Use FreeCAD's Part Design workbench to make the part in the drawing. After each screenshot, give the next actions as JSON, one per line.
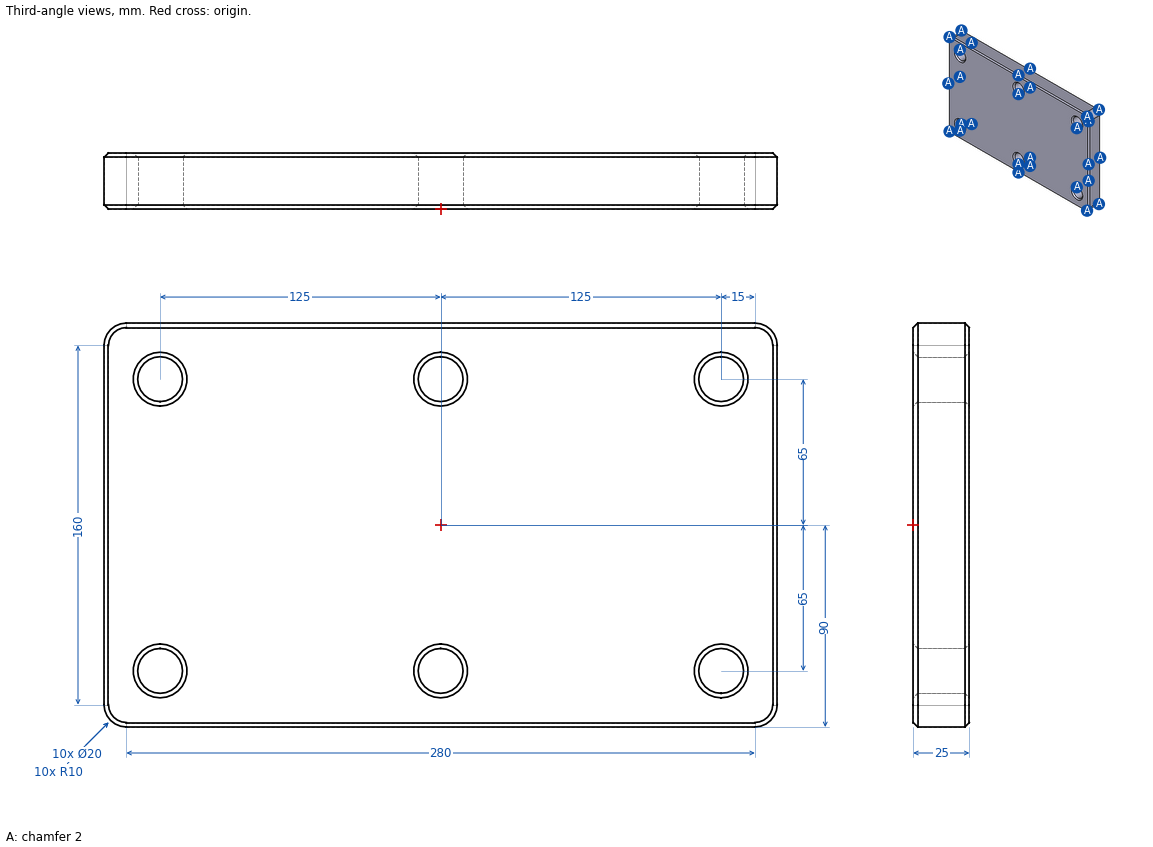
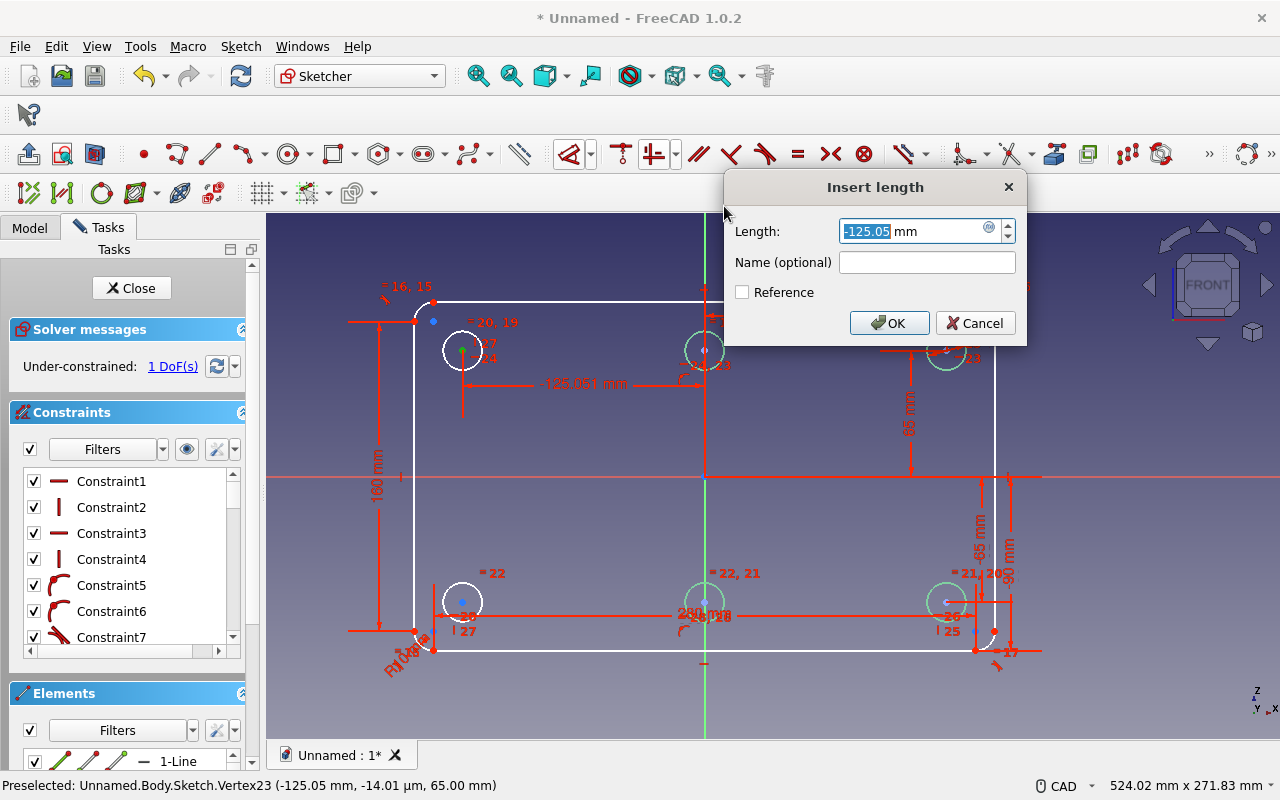
{"action": "type", "text": "-125"}
{"action": "key", "text": "Return"}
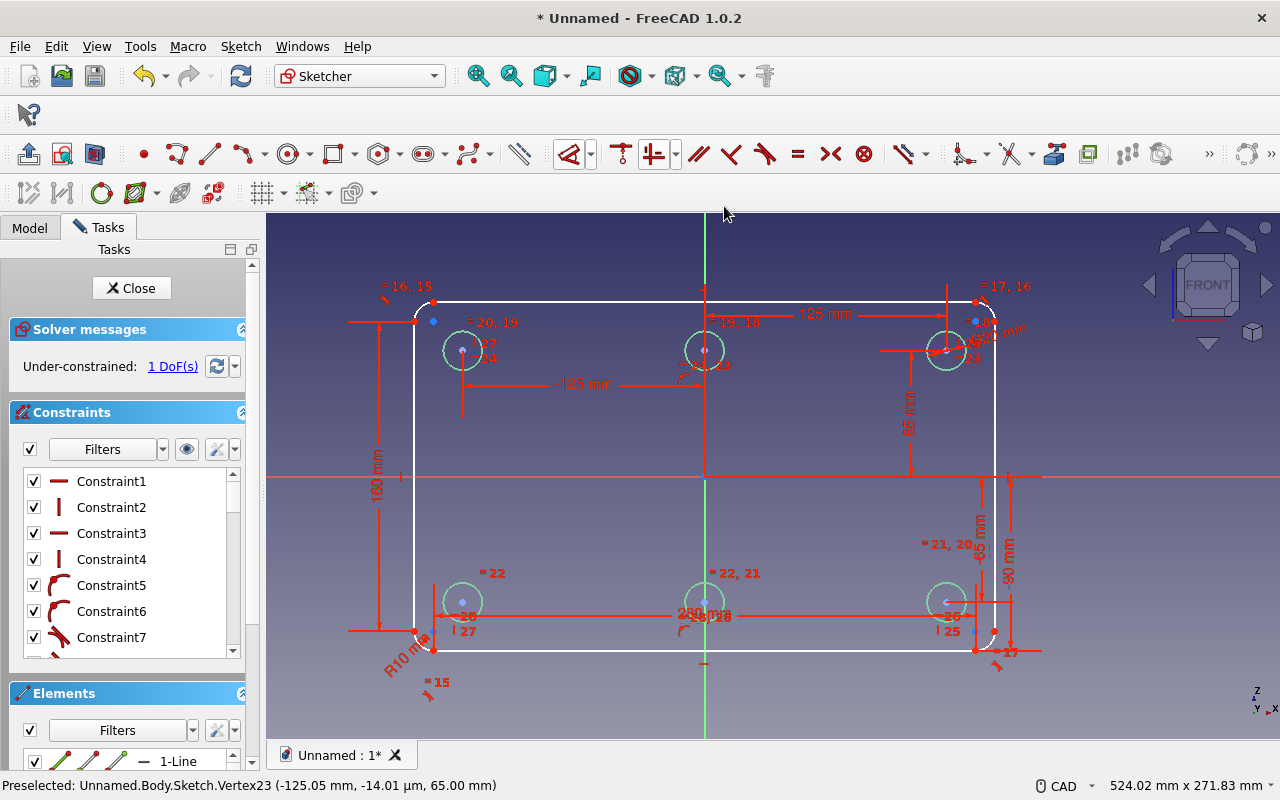
{"action": "scroll", "coordinate": [976, 302], "scroll_direction": "up", "scroll_amount": 2}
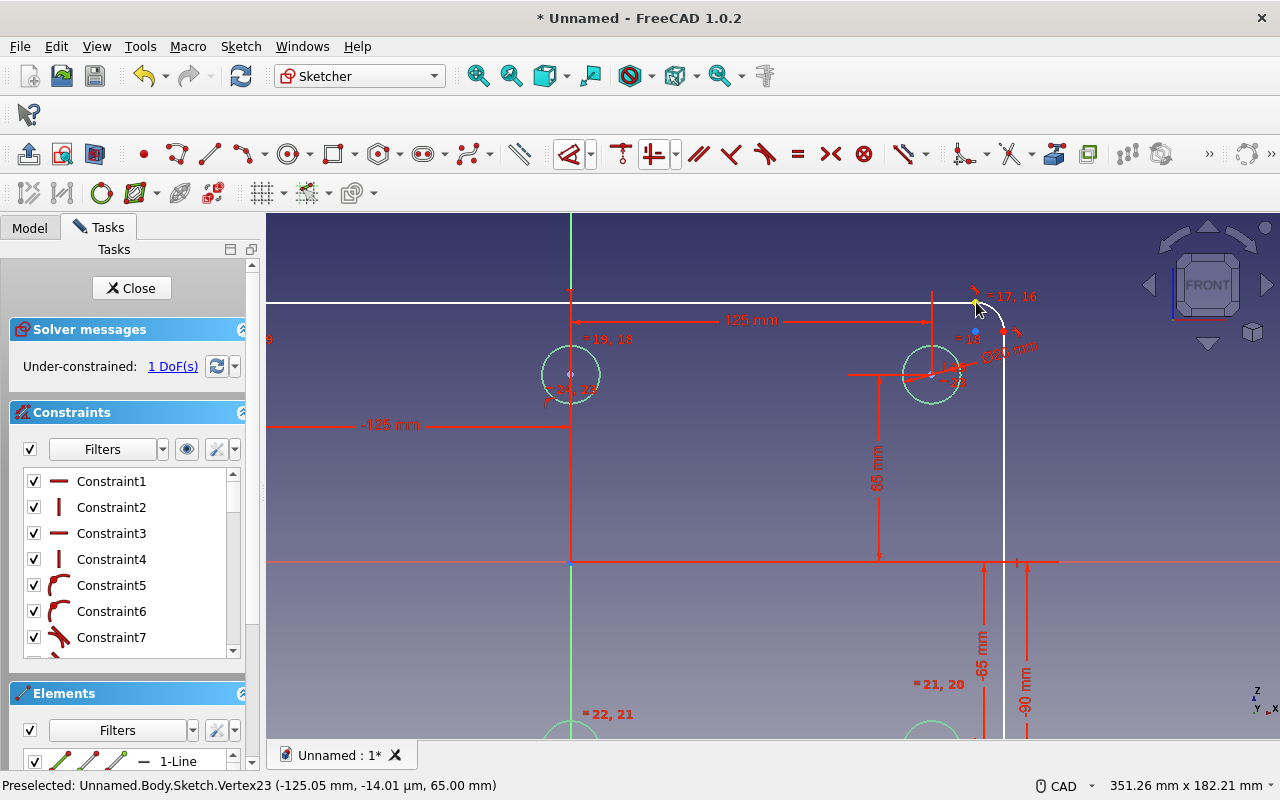
{"action": "left_click", "coordinate": [975, 303]}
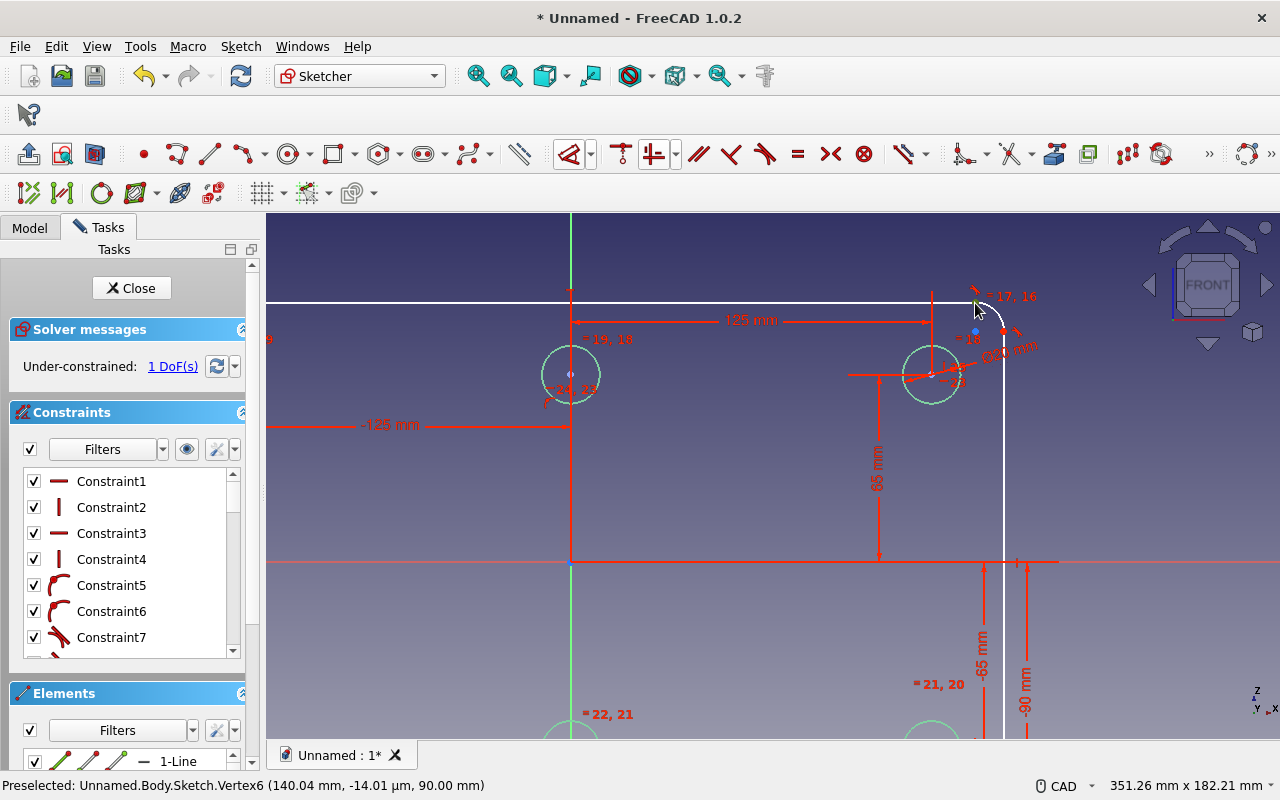
{"action": "left_click", "coordinate": [932, 375]}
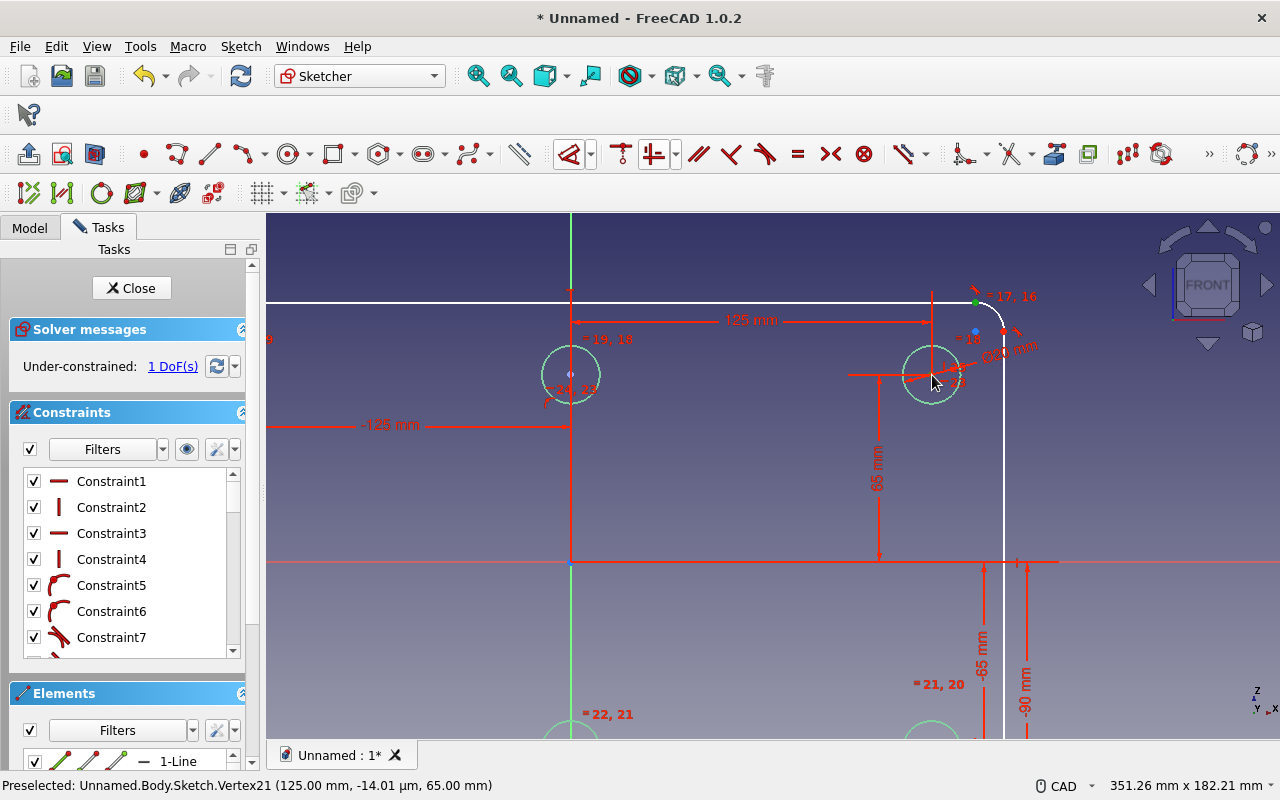
{"action": "key", "text": "l"}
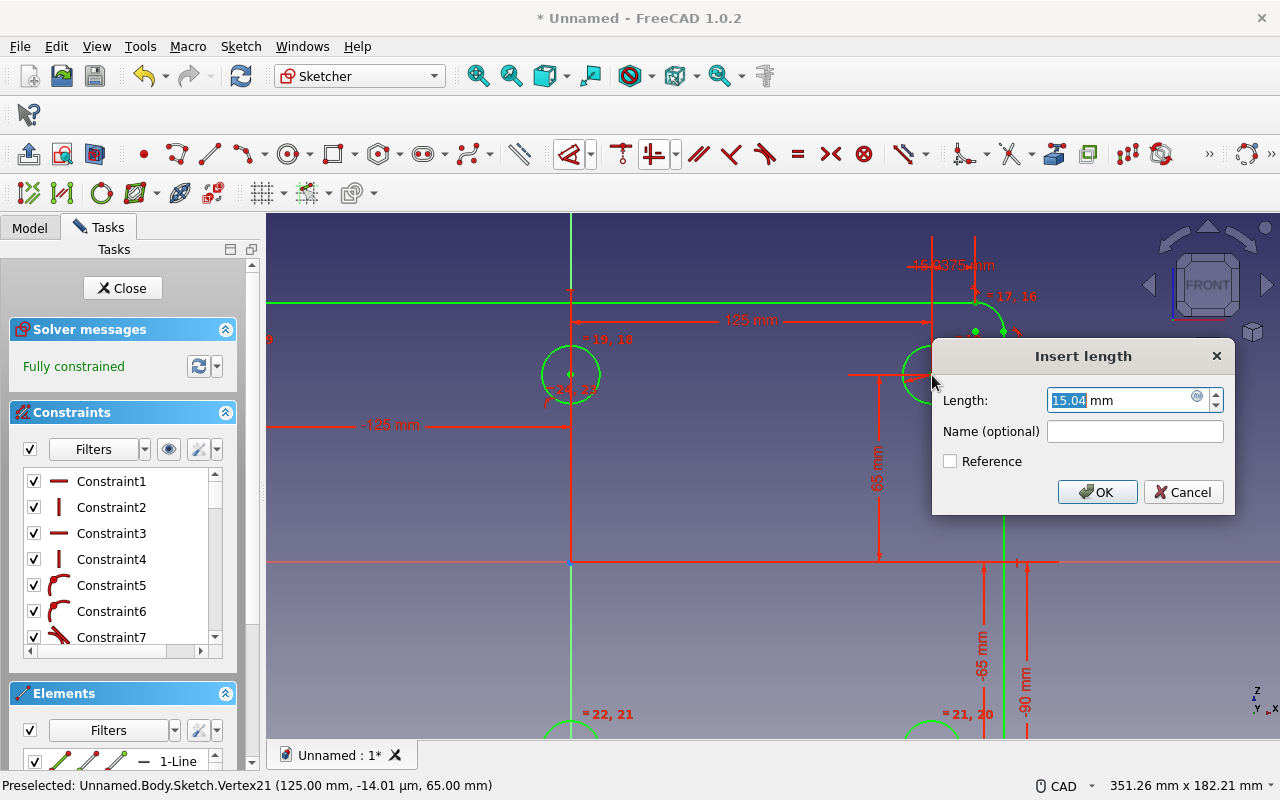
{"action": "type", "text": "15"}
{"action": "key", "text": "Return"}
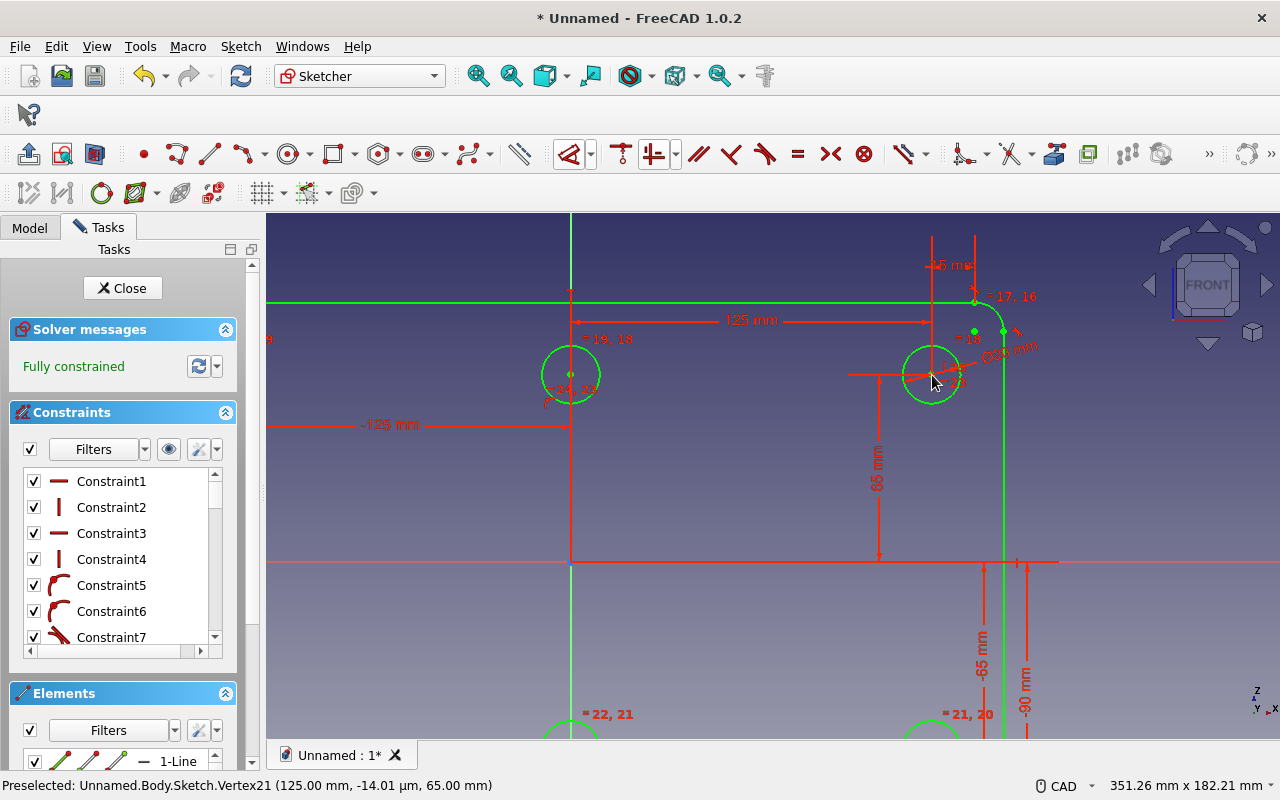
{"action": "left_click", "coordinate": [123, 288]}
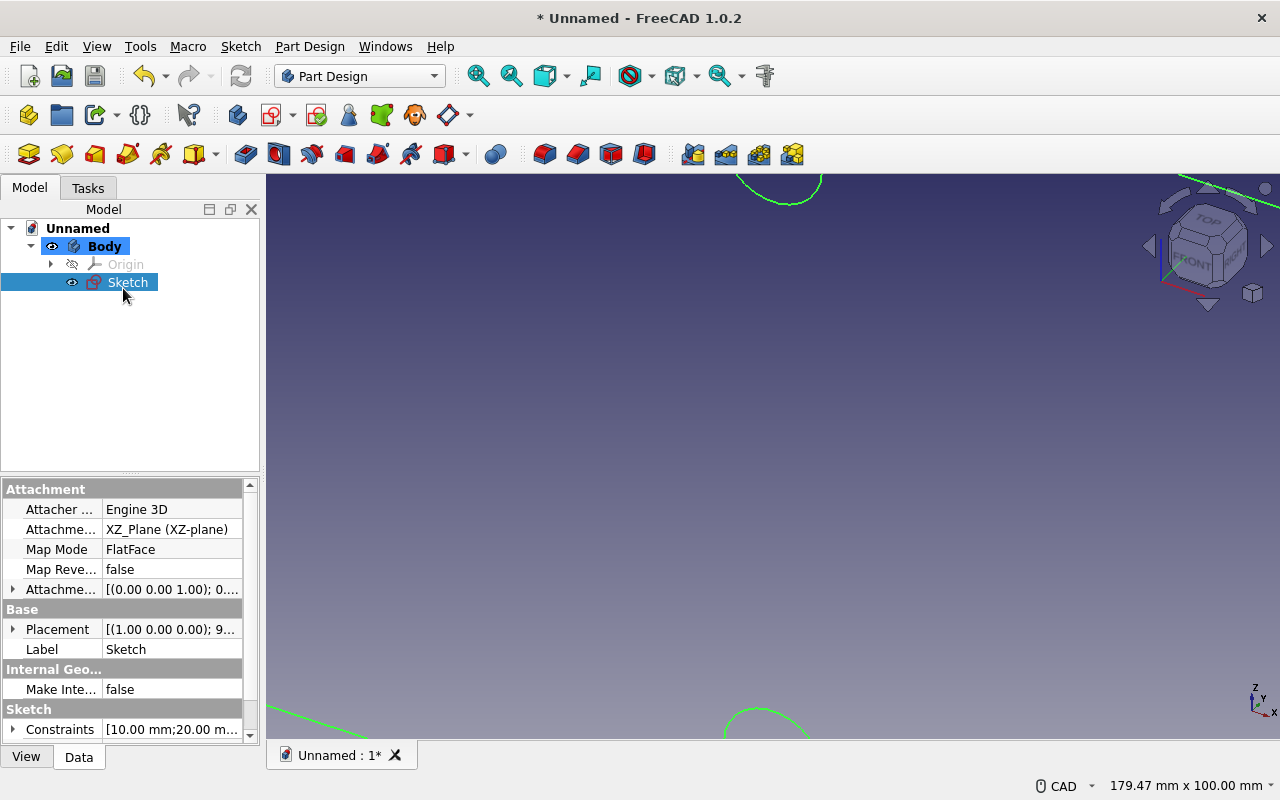
{"action": "left_click", "coordinate": [29, 154]}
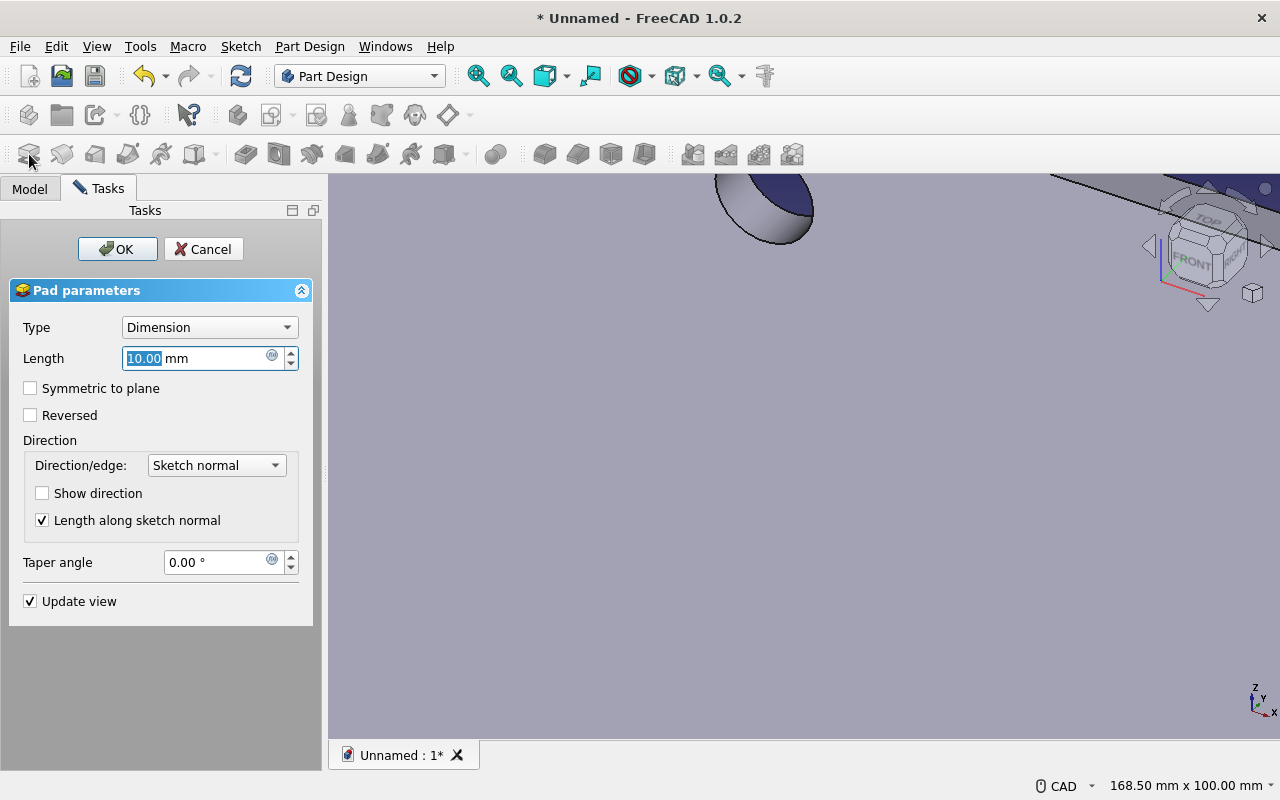
{"action": "type", "text": "25"}
{"action": "key", "text": "Tab"}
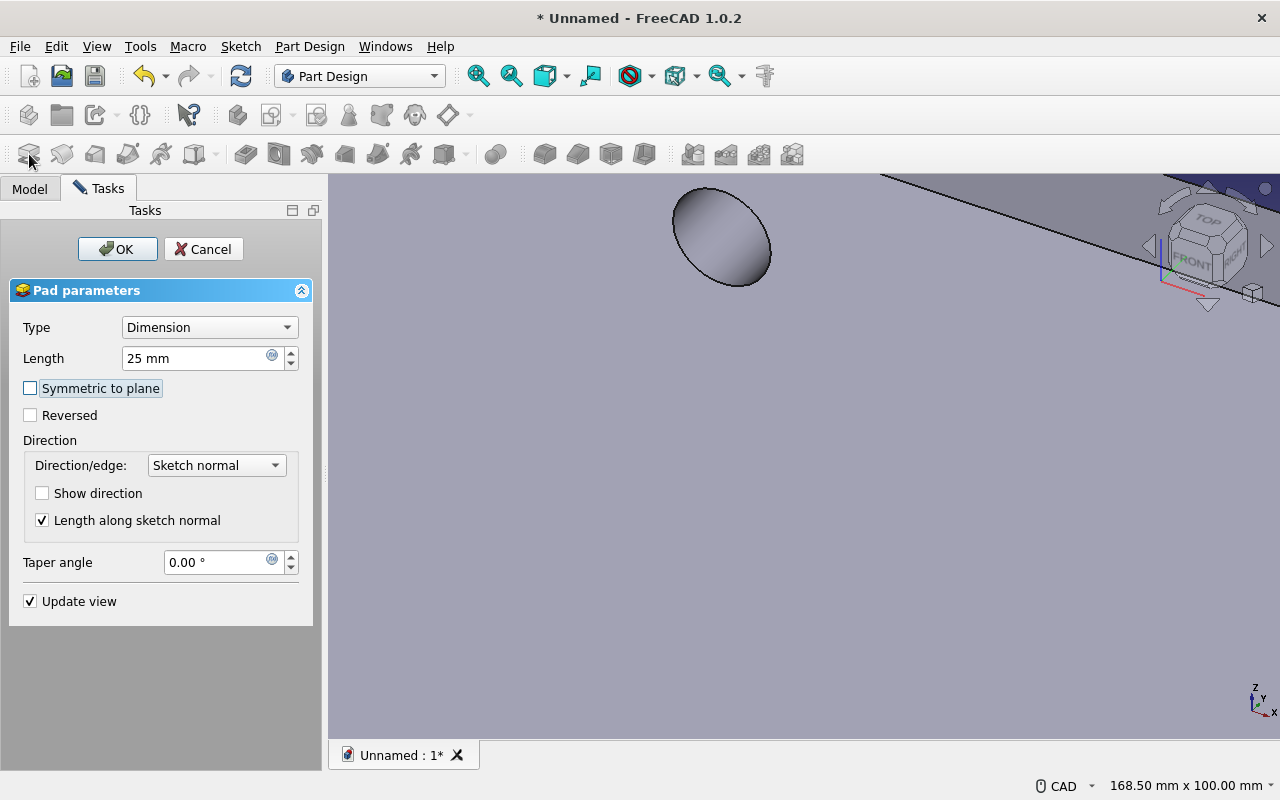
{"action": "left_click", "coordinate": [31, 415]}